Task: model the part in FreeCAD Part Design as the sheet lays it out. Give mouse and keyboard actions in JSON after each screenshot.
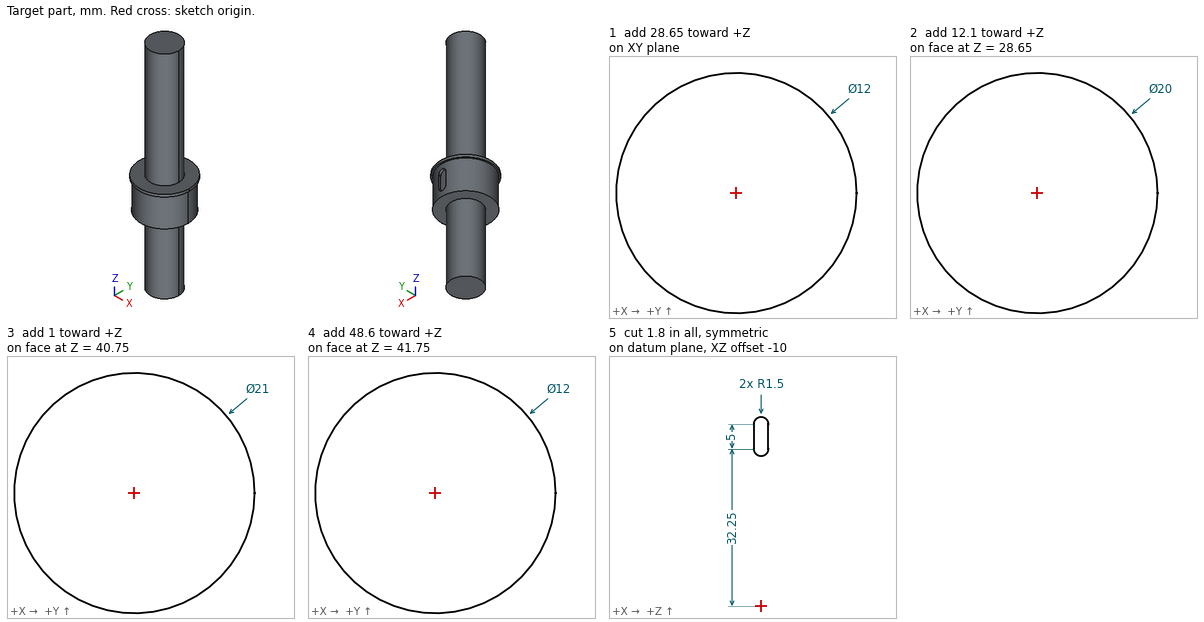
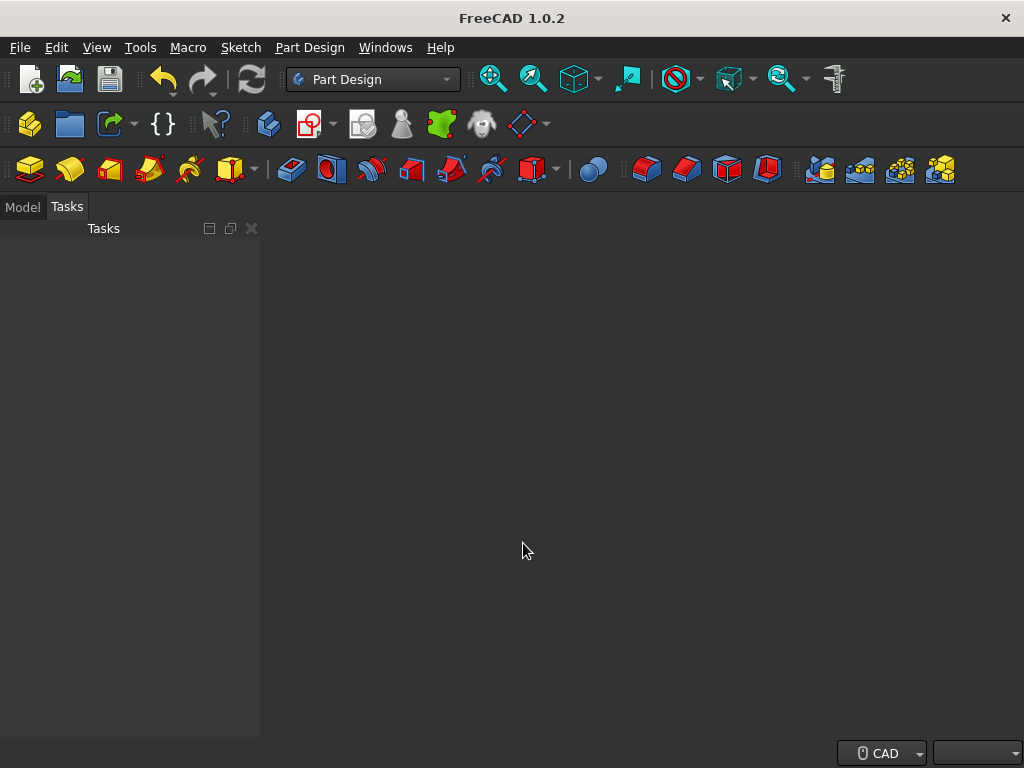
{"action": "left_click", "coordinate": [30, 80]}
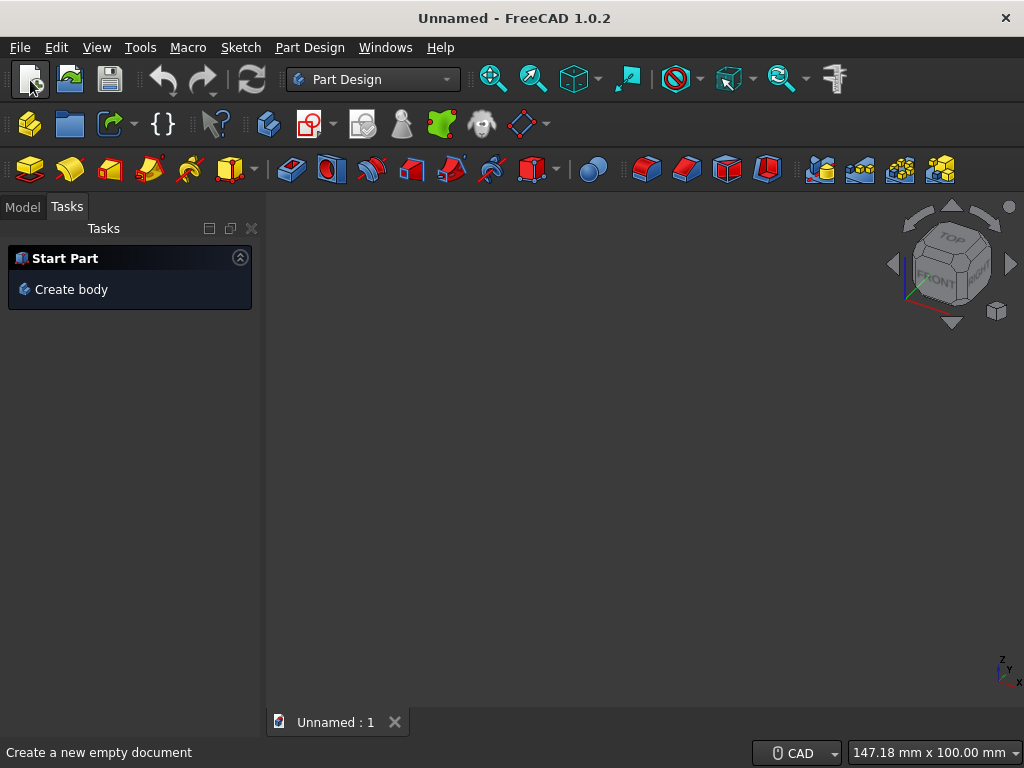
{"action": "left_click", "coordinate": [310, 124]}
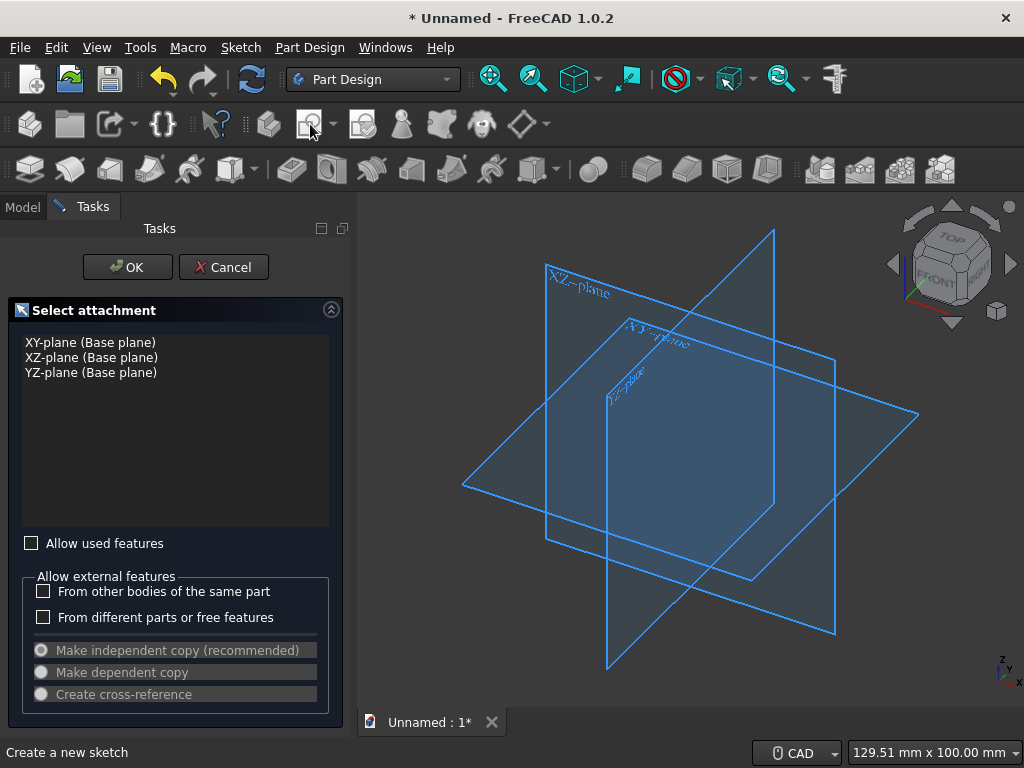
{"action": "left_click", "coordinate": [82, 342]}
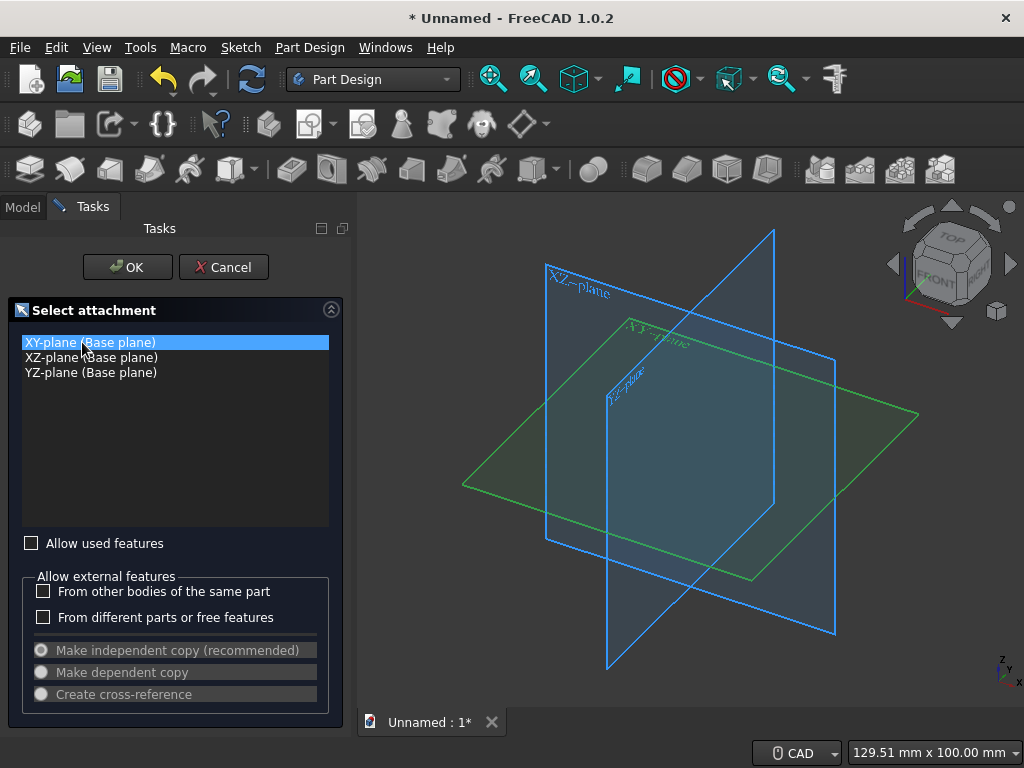
{"action": "left_click", "coordinate": [128, 267]}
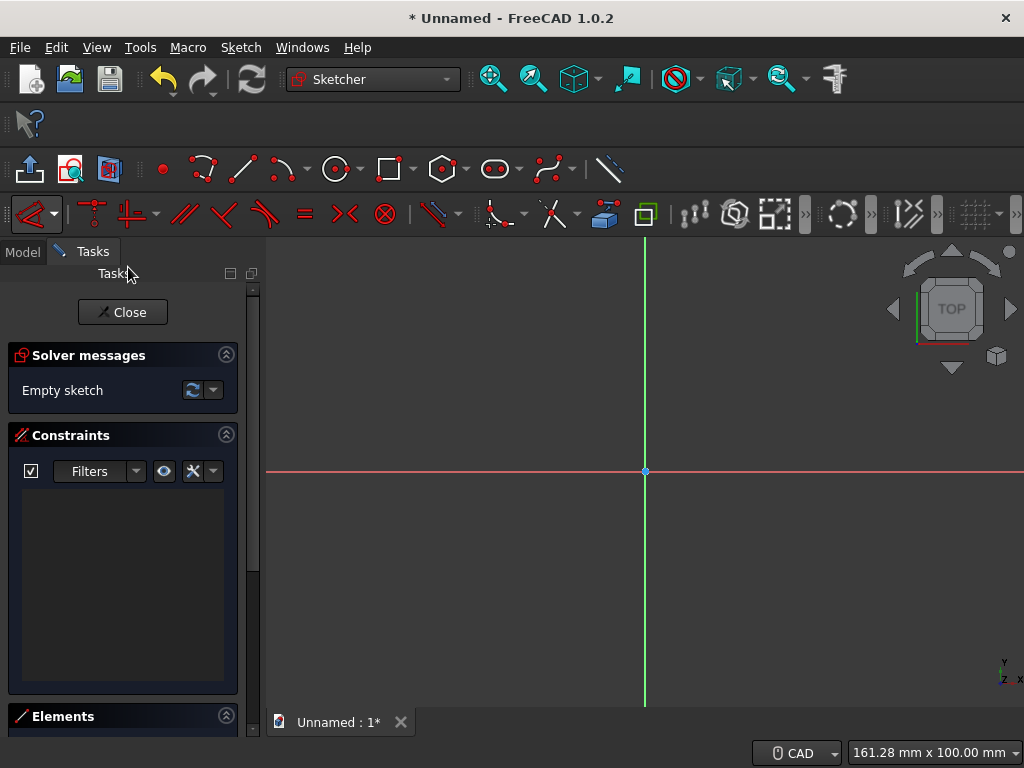
{"action": "scroll", "coordinate": [662, 472], "scroll_direction": "up", "scroll_amount": 8}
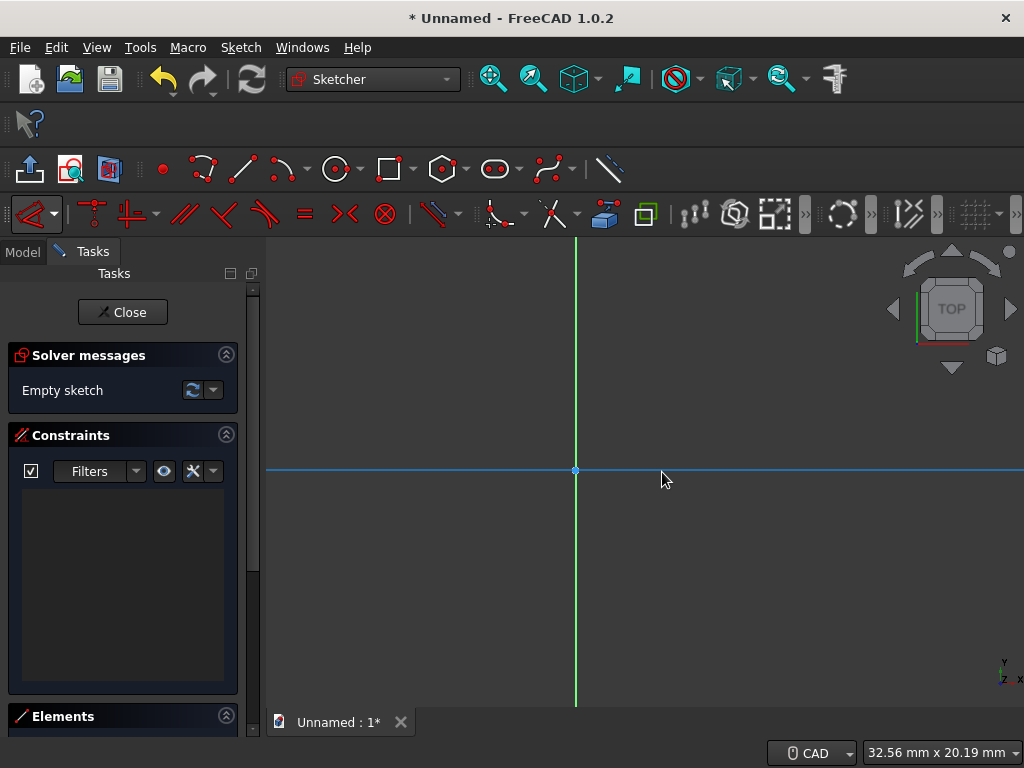
{"action": "left_click", "coordinate": [336, 170]}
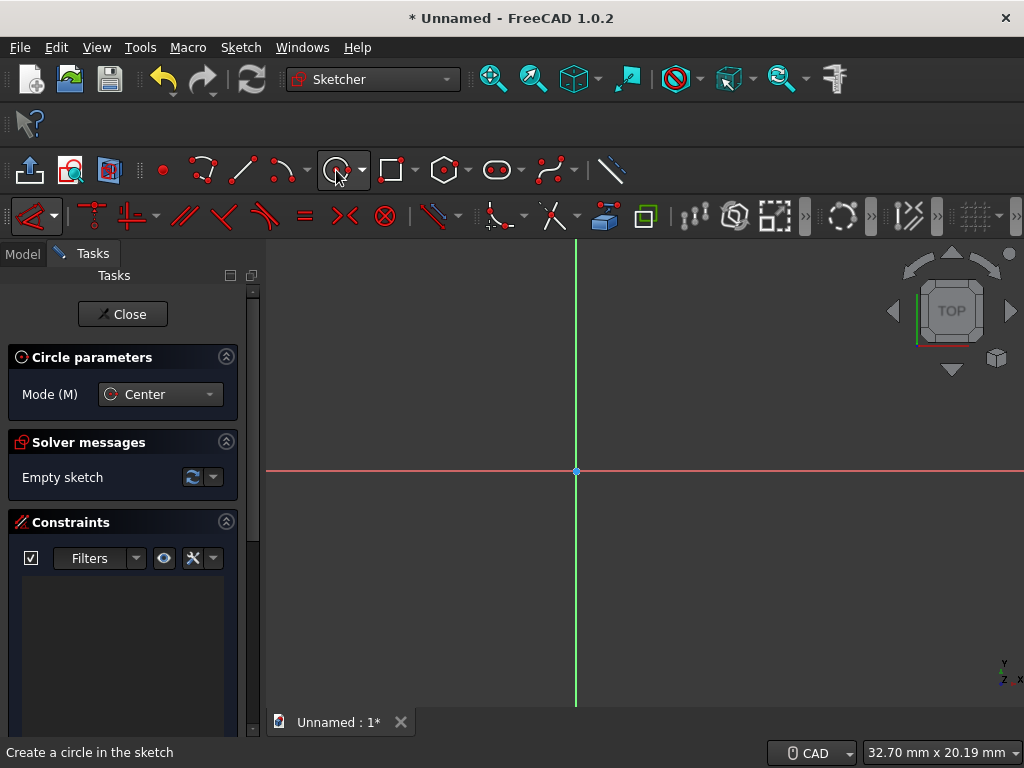
{"action": "left_click", "coordinate": [576, 471]}
{"action": "left_click", "coordinate": [674, 373]}
{"action": "key", "text": "Escape"}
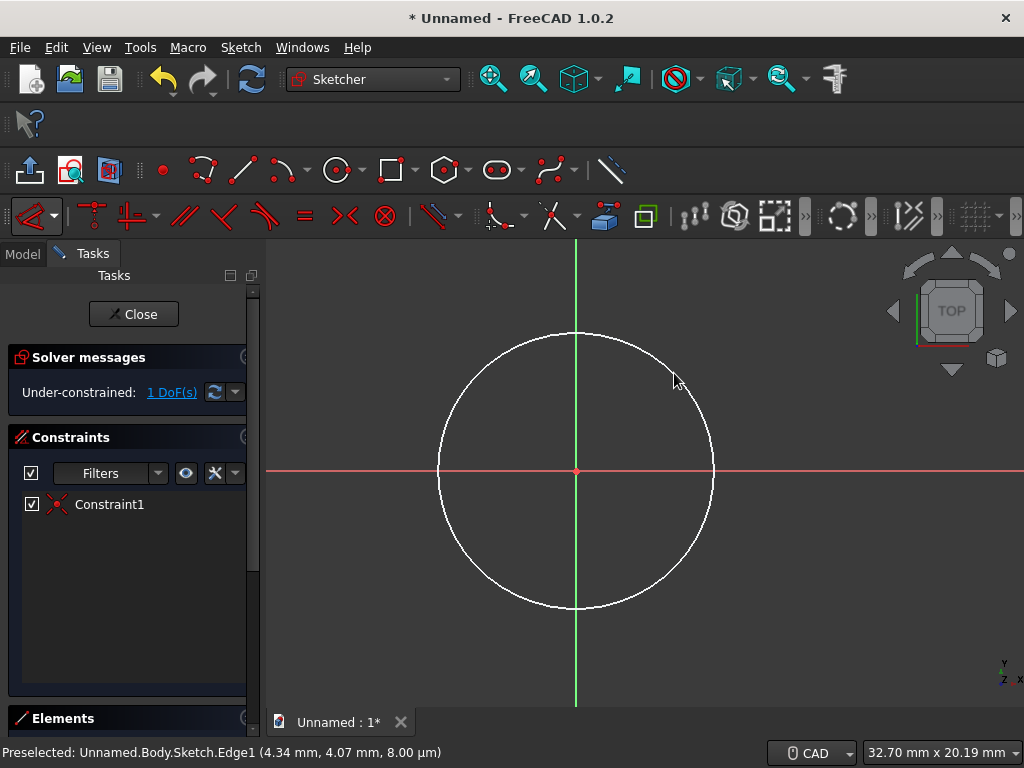
{"action": "left_click", "coordinate": [673, 373]}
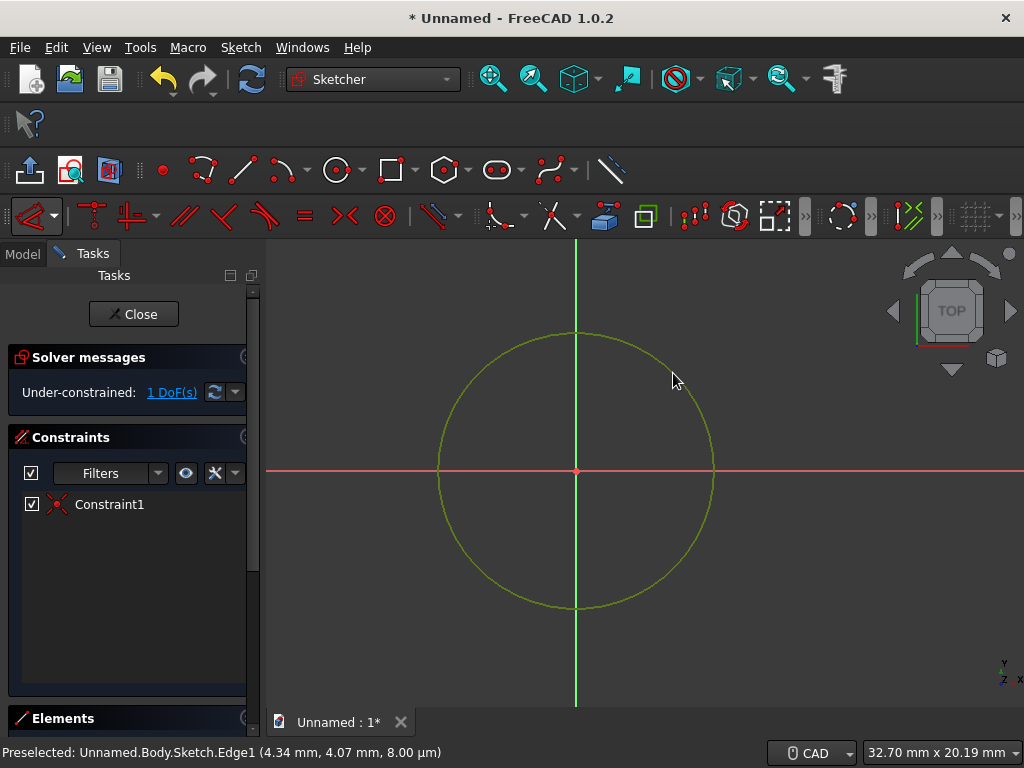
{"action": "key", "text": "k o"}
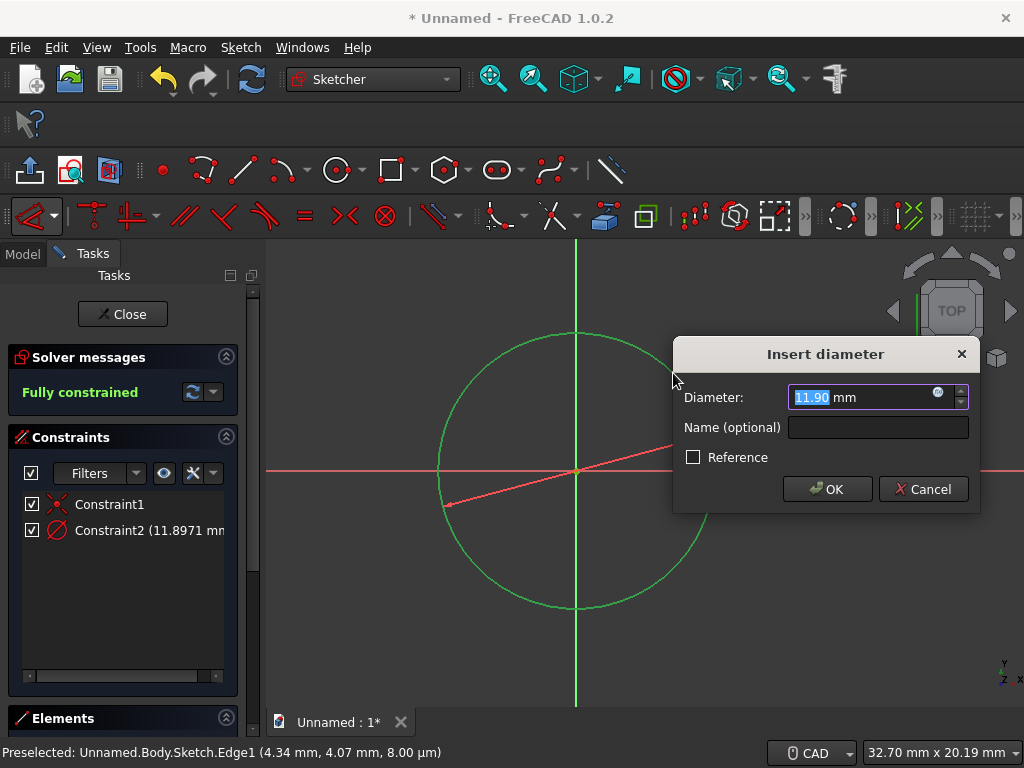
{"action": "type", "text": "12"}
{"action": "key", "text": "Return"}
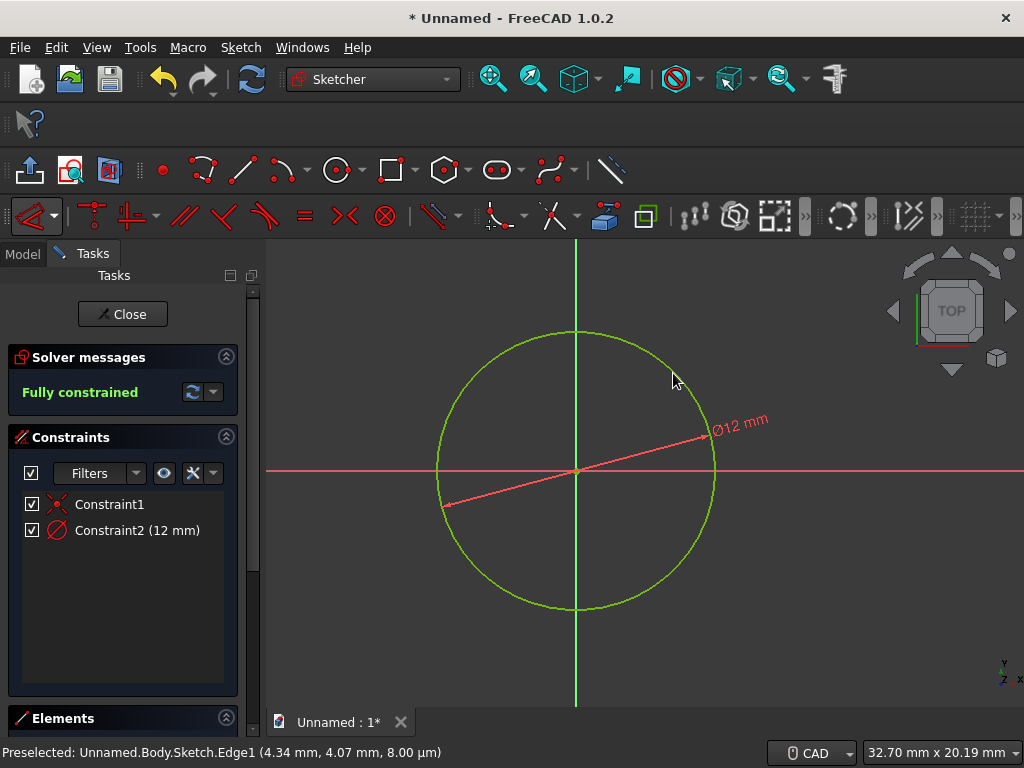
{"action": "left_click", "coordinate": [123, 314]}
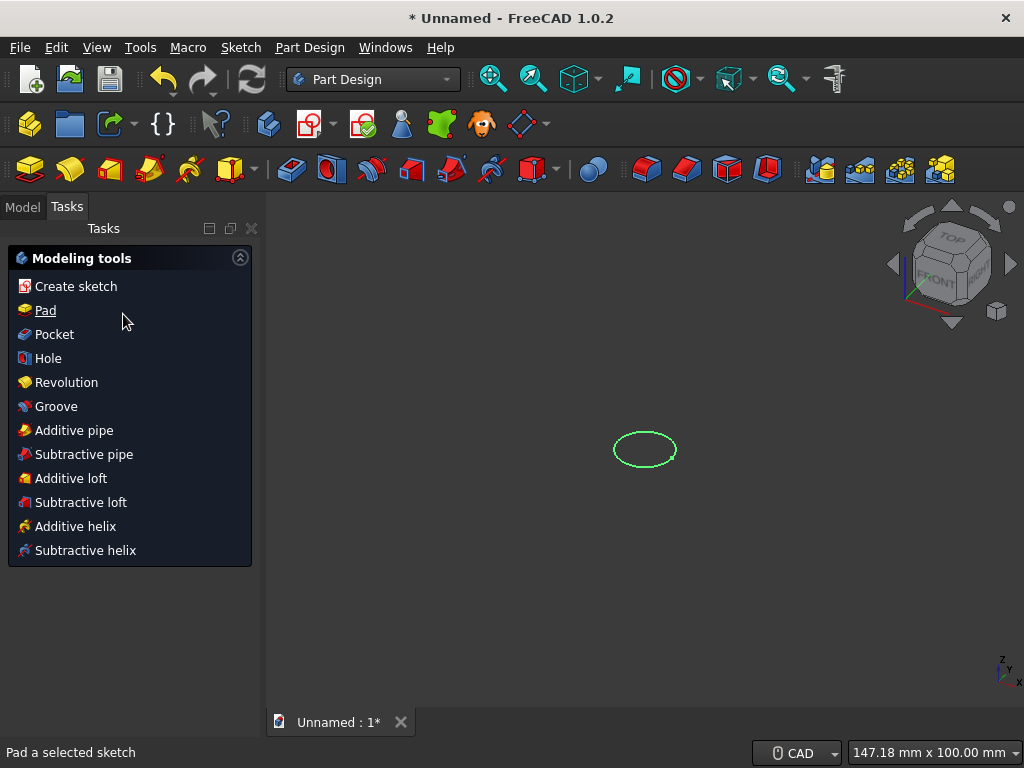
{"action": "left_click", "coordinate": [30, 170]}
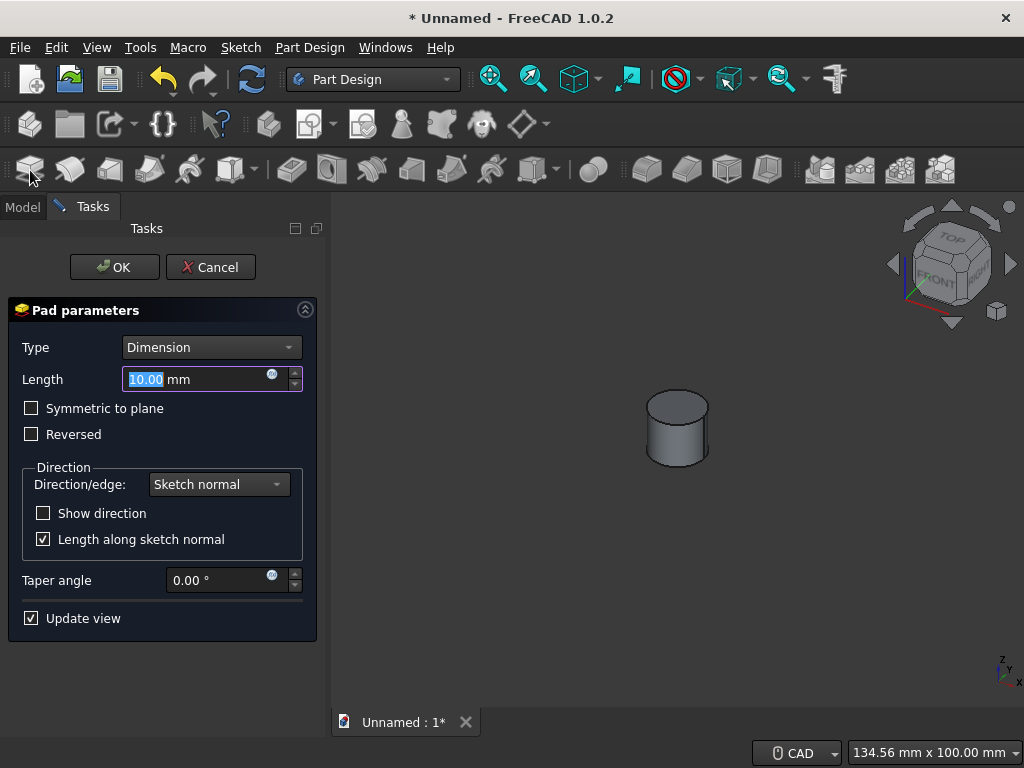
{"action": "type", "text": "28.65"}
{"action": "key", "text": "Tab"}